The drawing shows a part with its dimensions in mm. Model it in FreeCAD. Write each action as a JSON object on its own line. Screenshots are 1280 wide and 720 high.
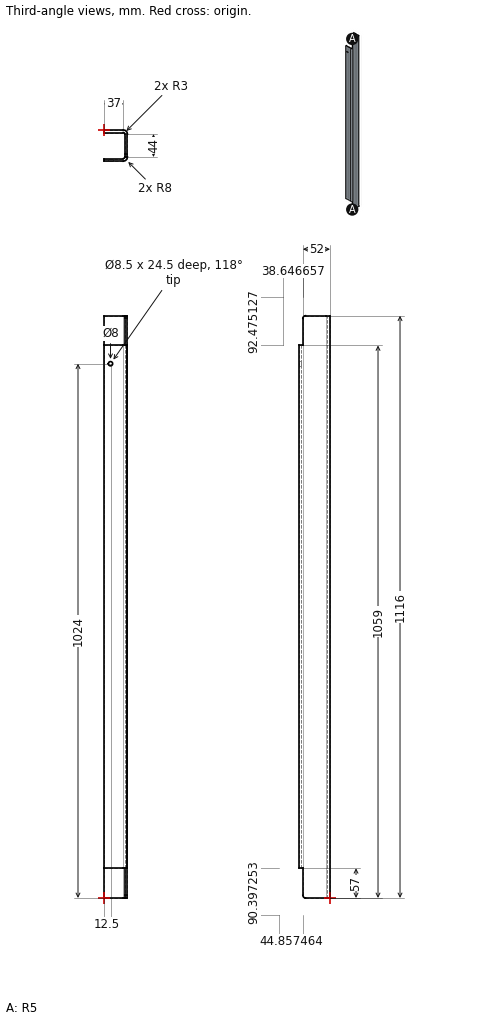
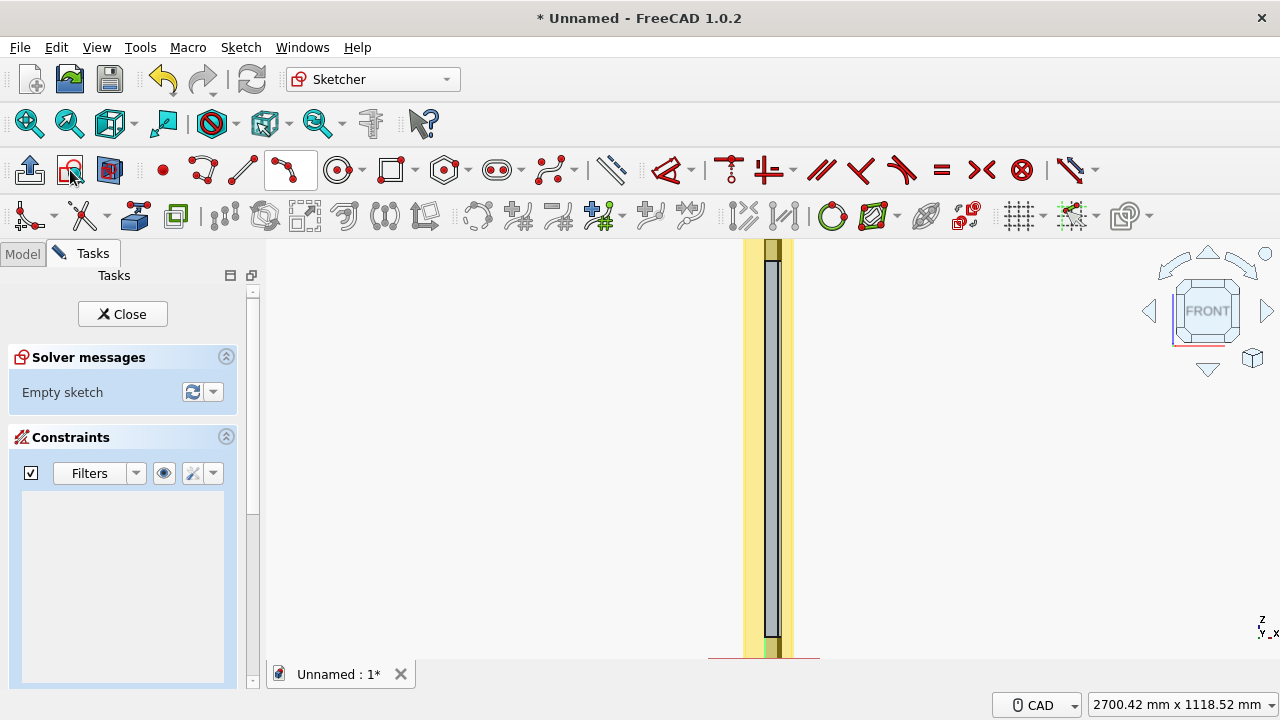
{"action": "key", "text": "q s"}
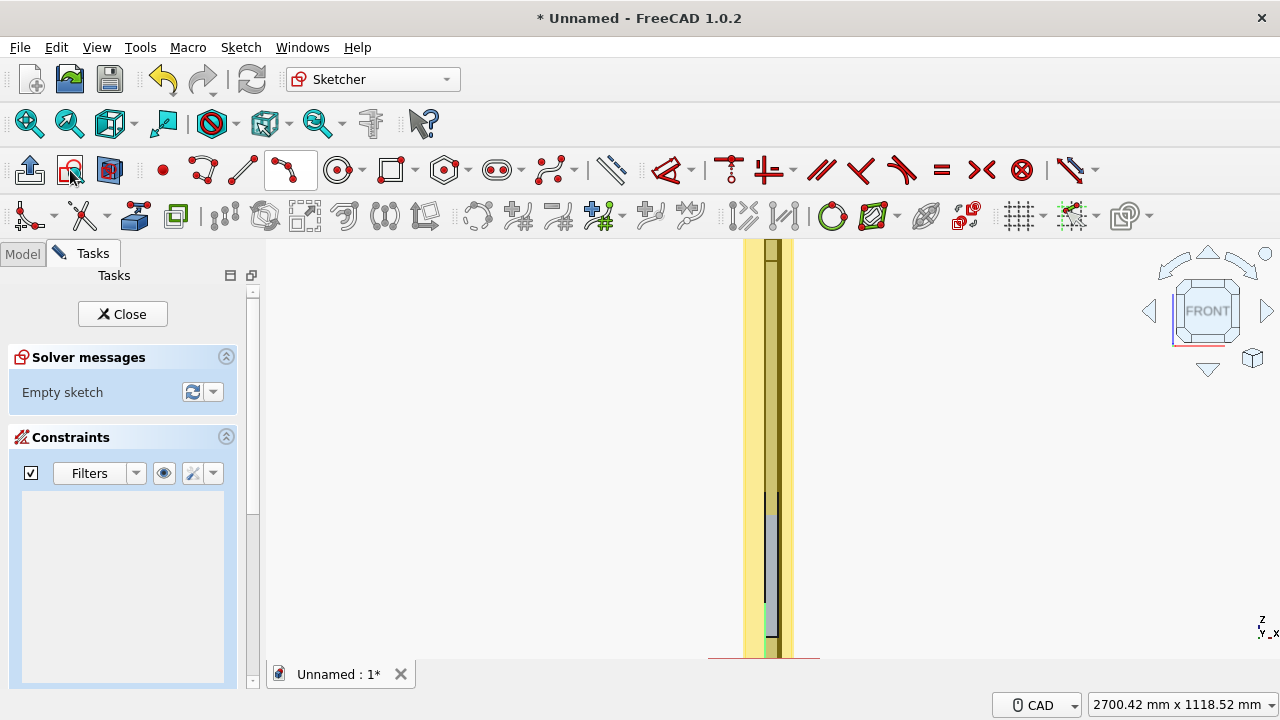
{"action": "scroll", "coordinate": [773, 267], "scroll_direction": "up", "scroll_amount": 15}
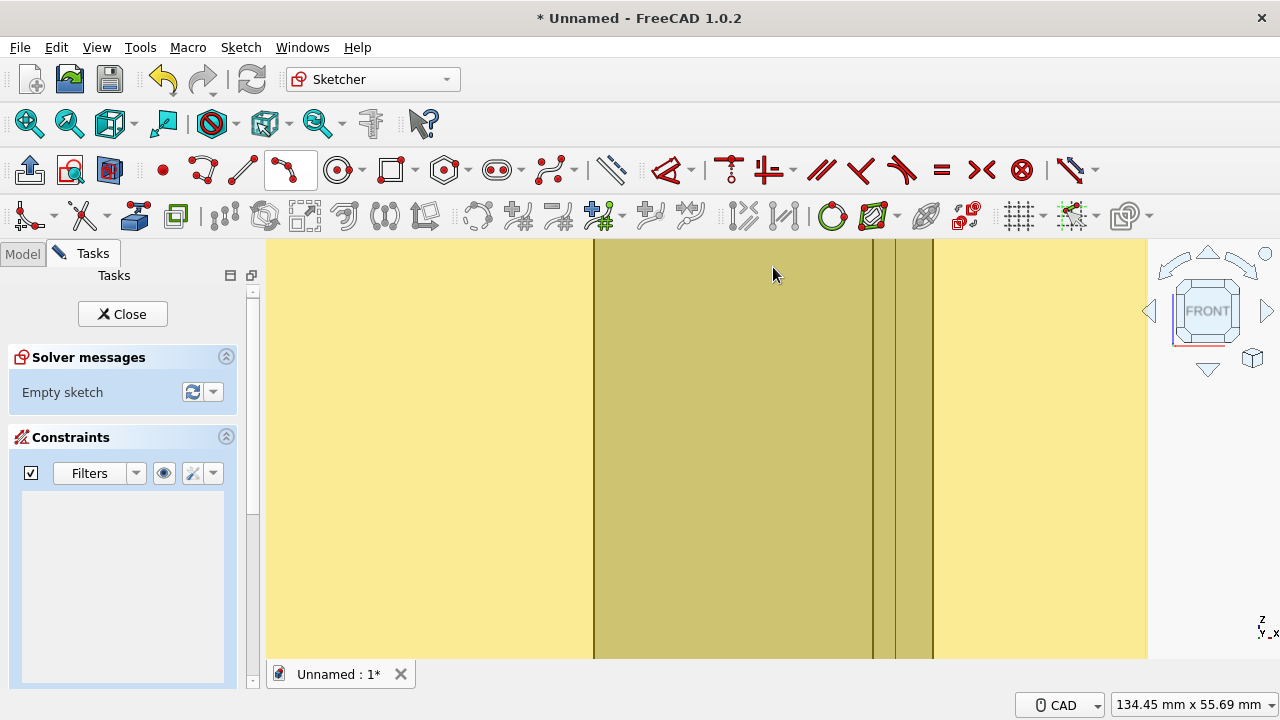
{"action": "scroll", "coordinate": [683, 393], "scroll_direction": "up", "scroll_amount": 7}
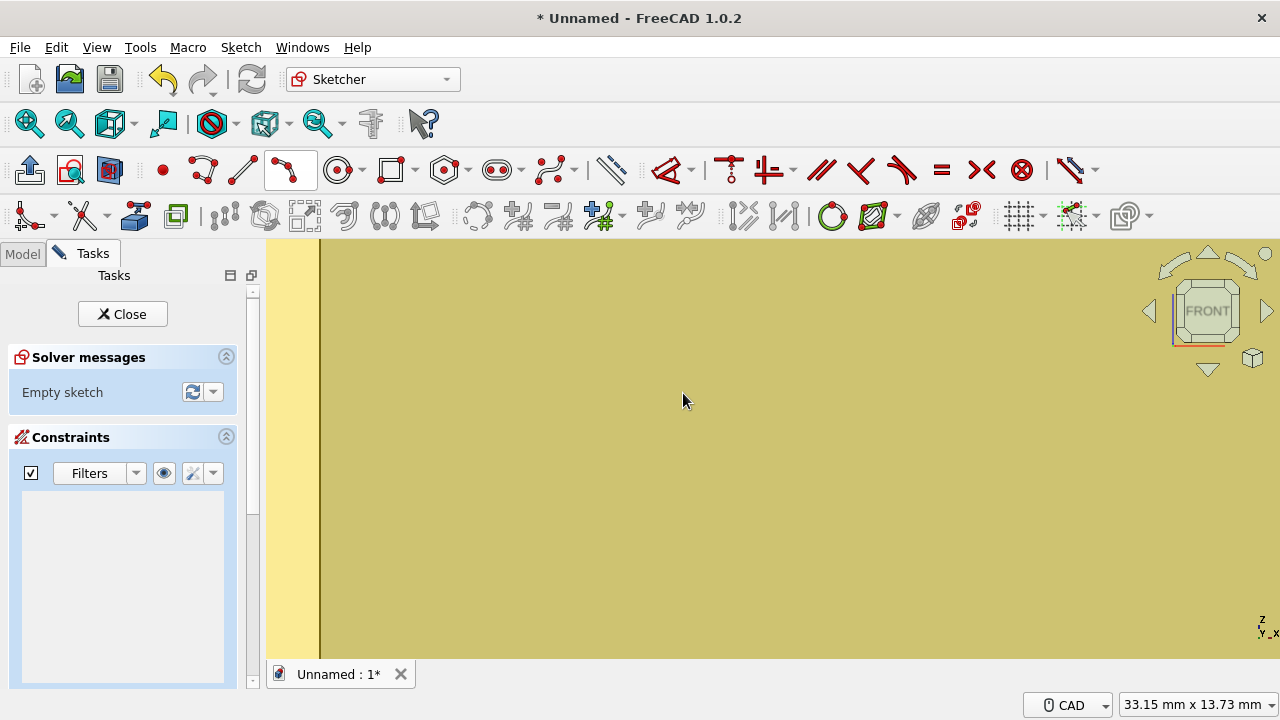
{"action": "key", "text": "g c"}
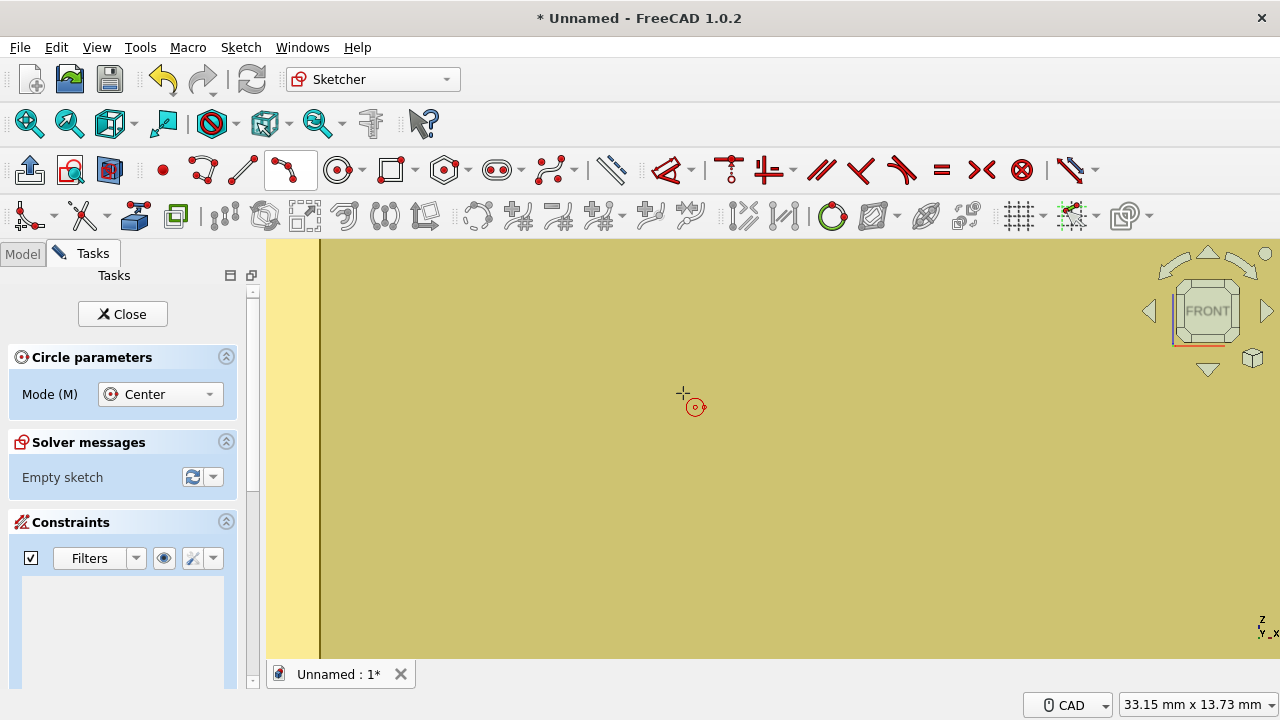
{"action": "left_click", "coordinate": [702, 447]}
{"action": "mouse_move", "coordinate": [789, 361]}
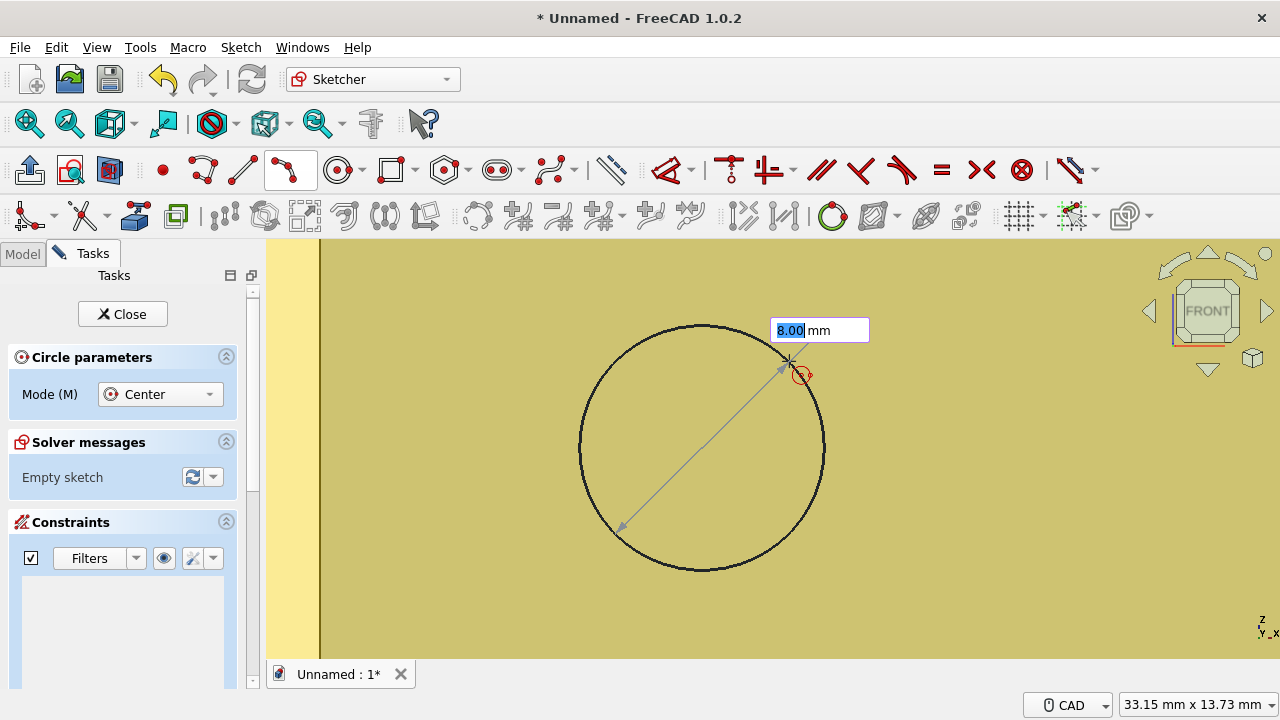
{"action": "type", "text": "8"}
{"action": "key", "text": "Return"}
{"action": "key", "text": "Escape"}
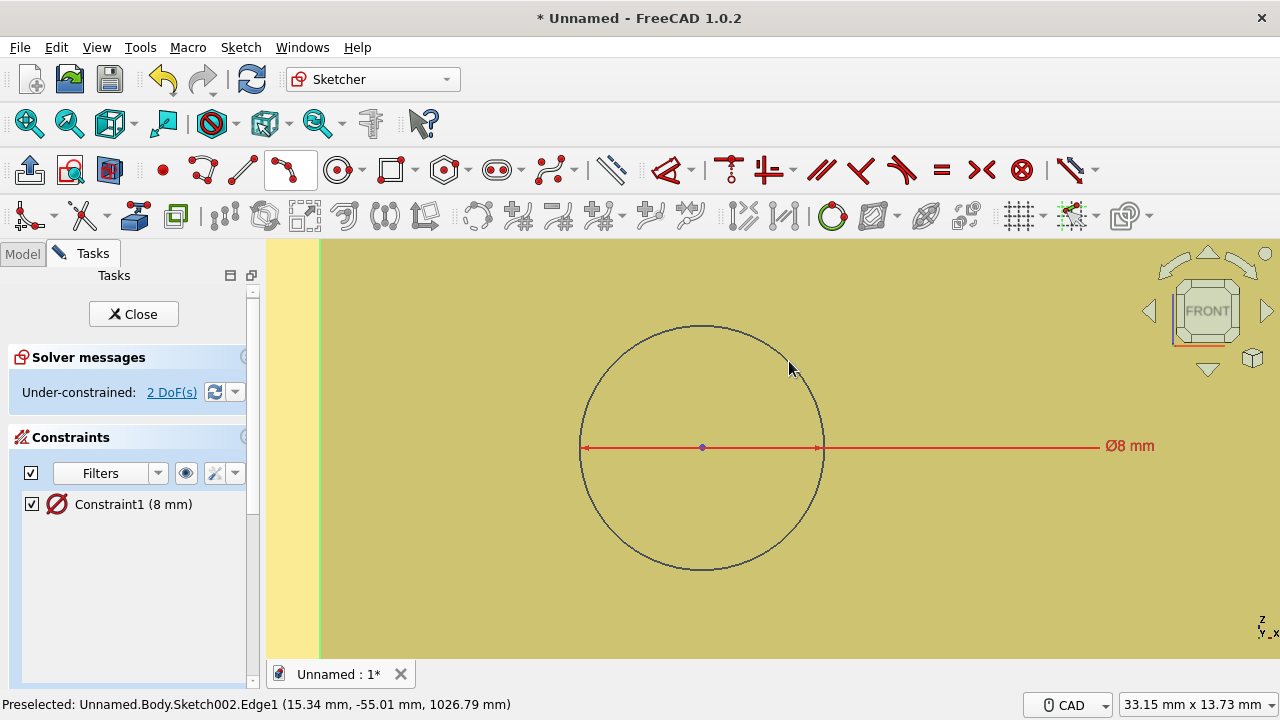
{"action": "key", "text": "d"}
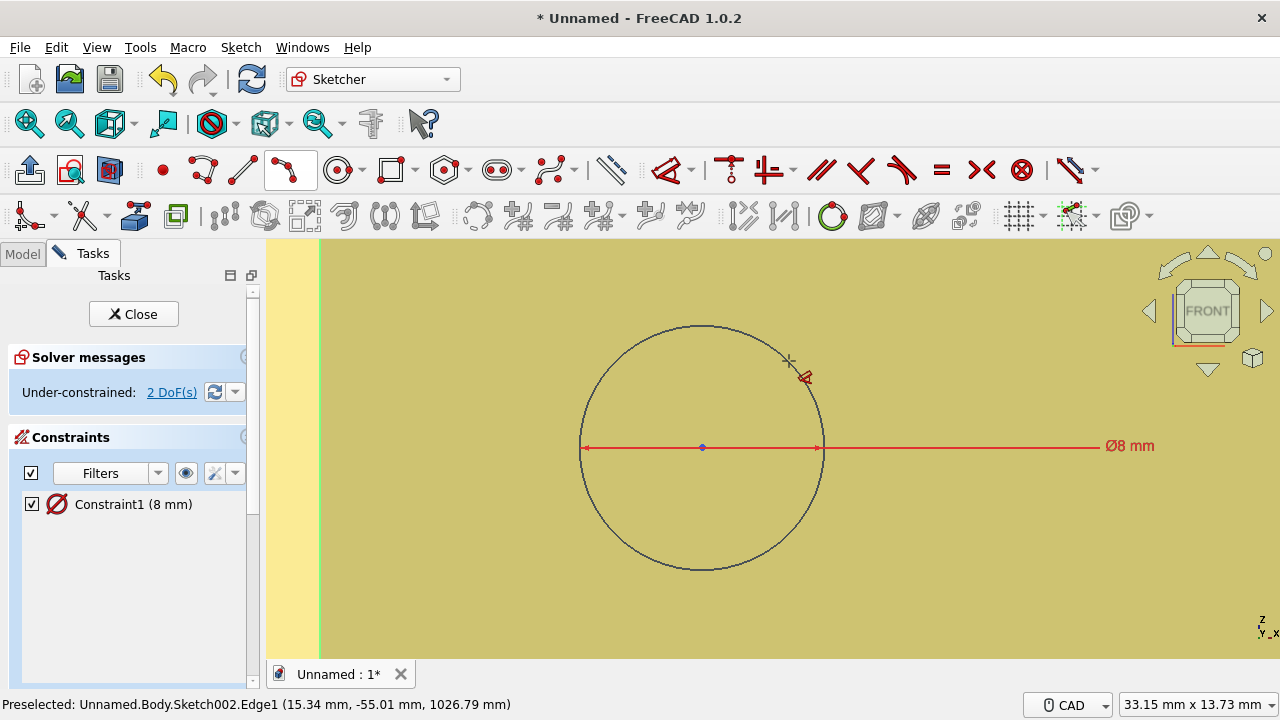
{"action": "left_click", "coordinate": [702, 448]}
{"action": "left_click", "coordinate": [511, 414]}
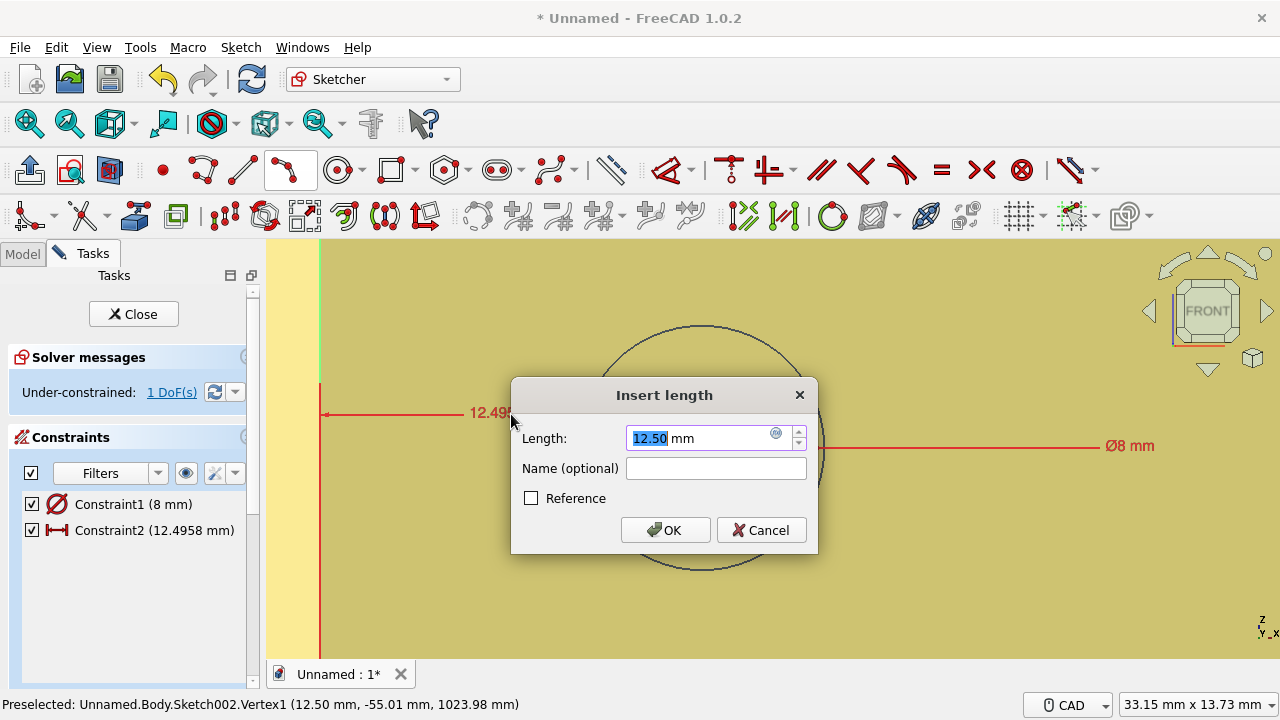
{"action": "type", "text": "12.5"}
{"action": "key", "text": "Return"}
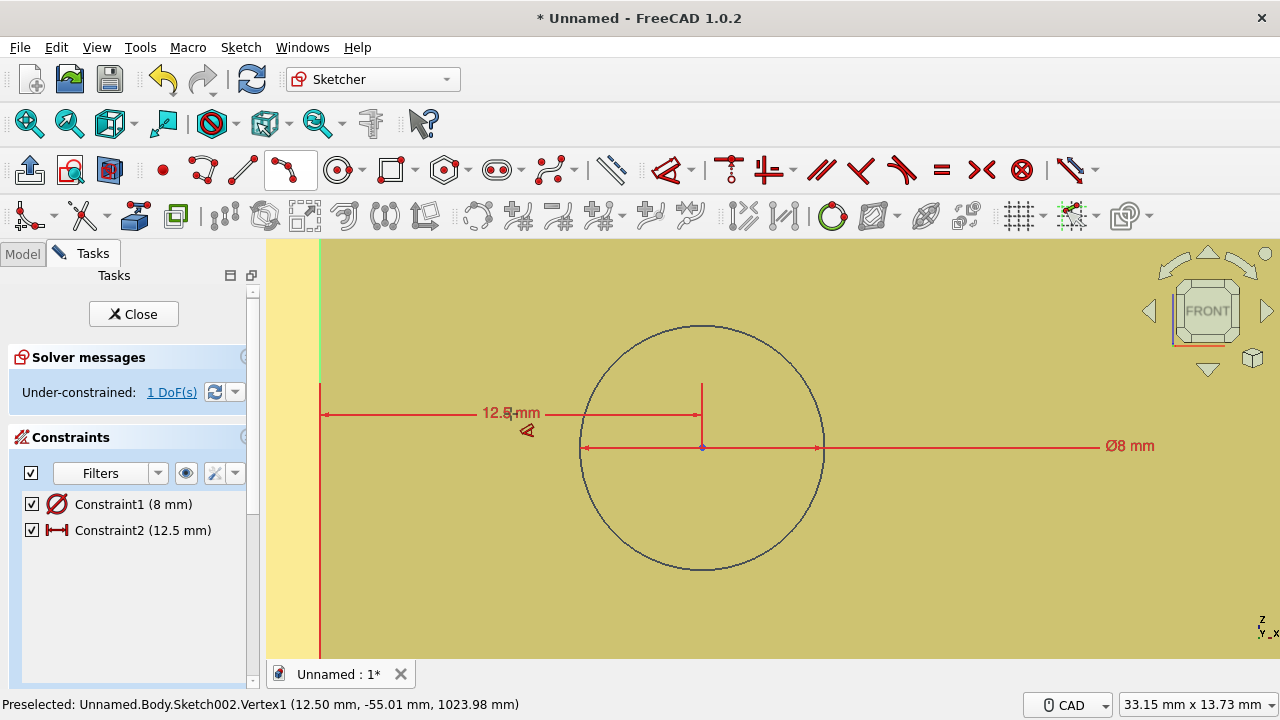
{"action": "left_click", "coordinate": [702, 448]}
{"action": "left_click", "coordinate": [736, 539]}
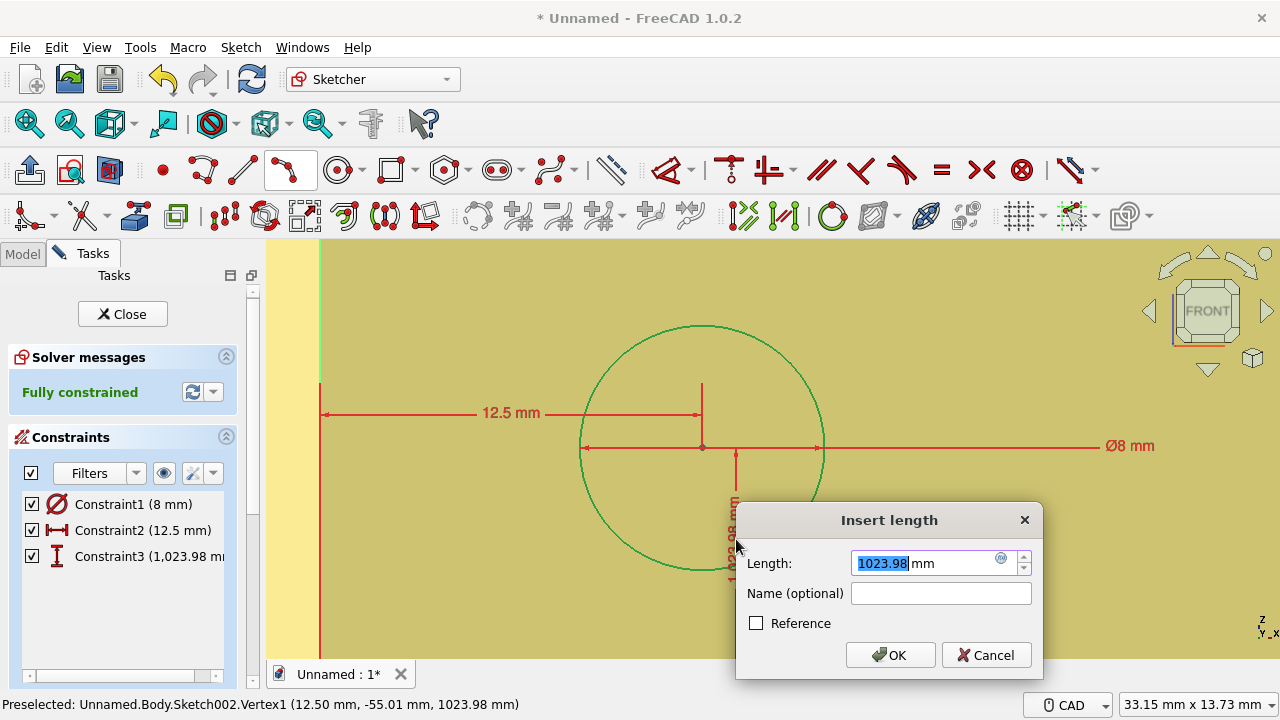
{"action": "type", "text": "1024"}
{"action": "key", "text": "Return"}
{"action": "key", "text": "Escape"}